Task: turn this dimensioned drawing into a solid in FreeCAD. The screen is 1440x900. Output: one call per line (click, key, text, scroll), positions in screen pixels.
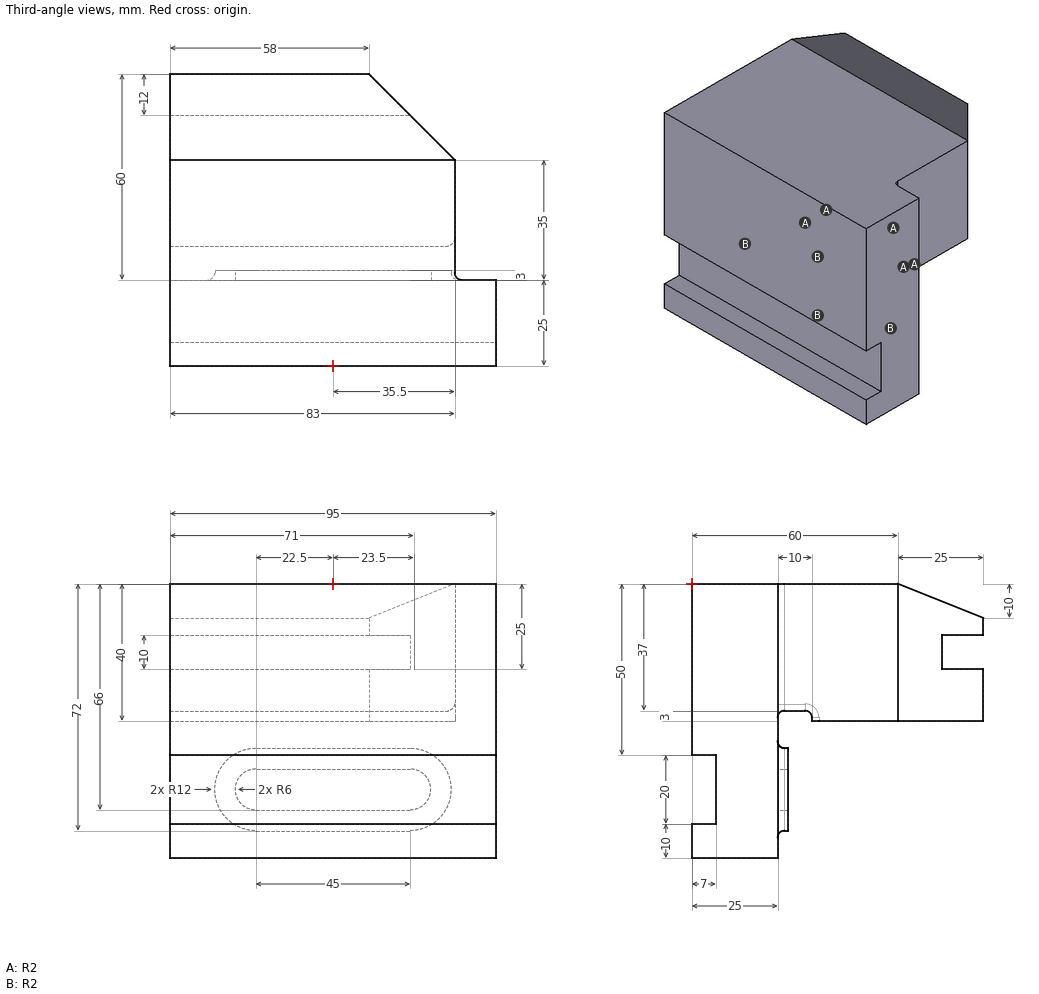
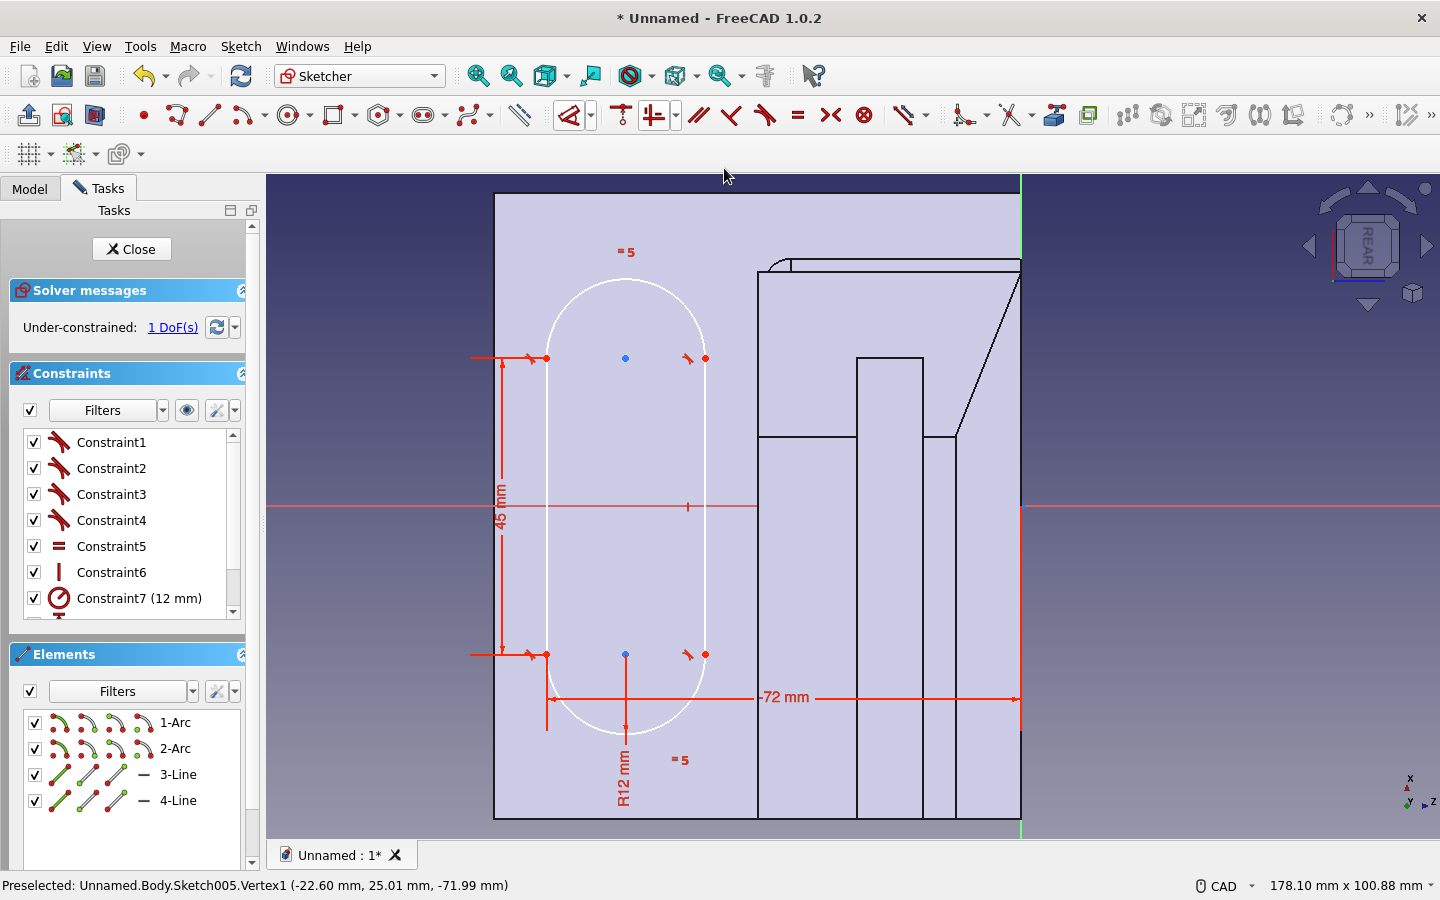
click(547, 655)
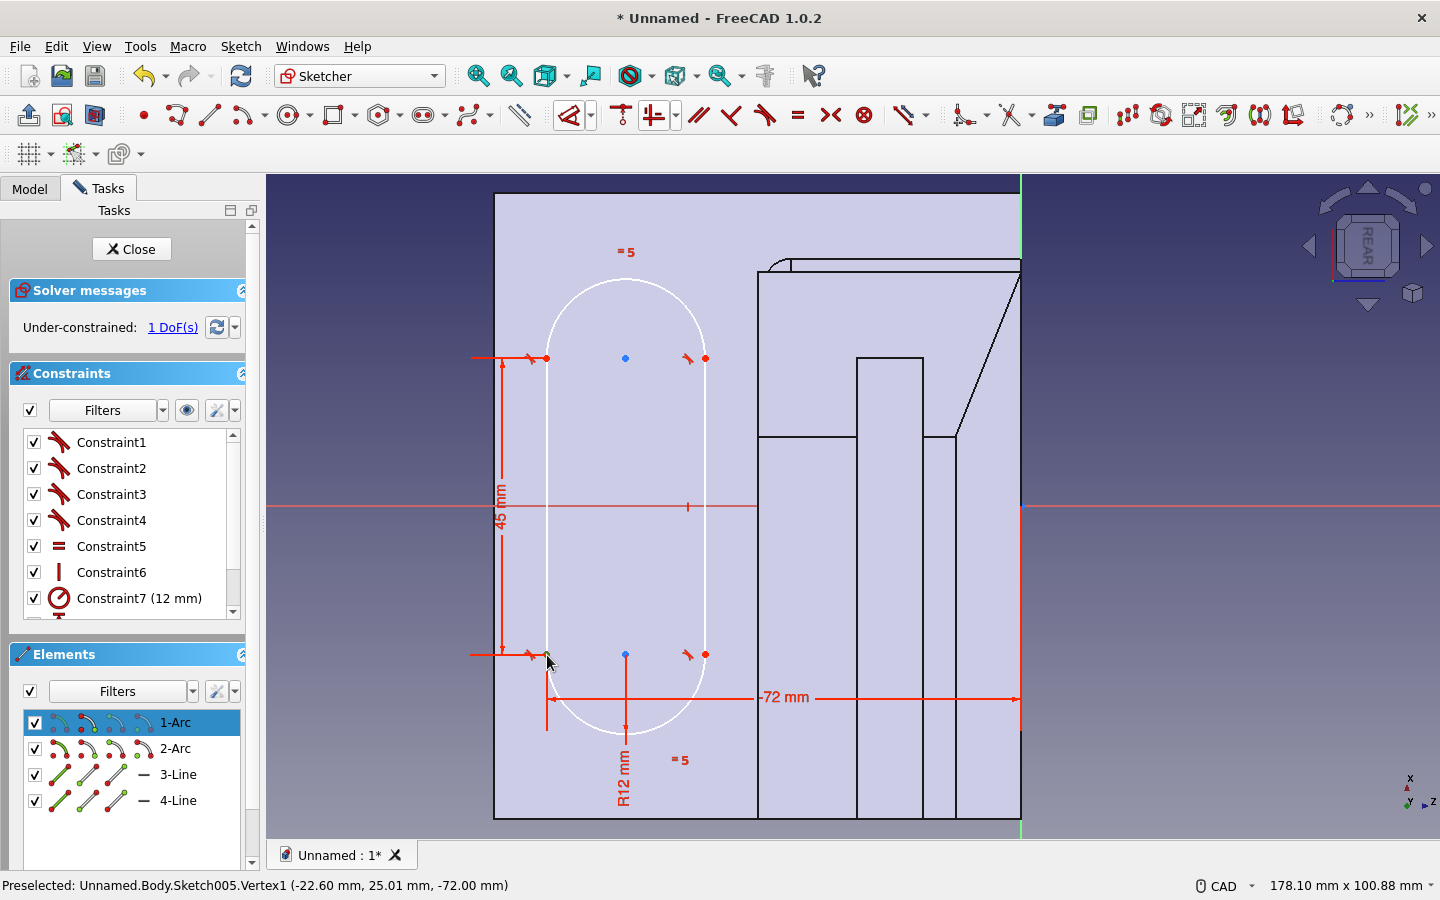
click(590, 116)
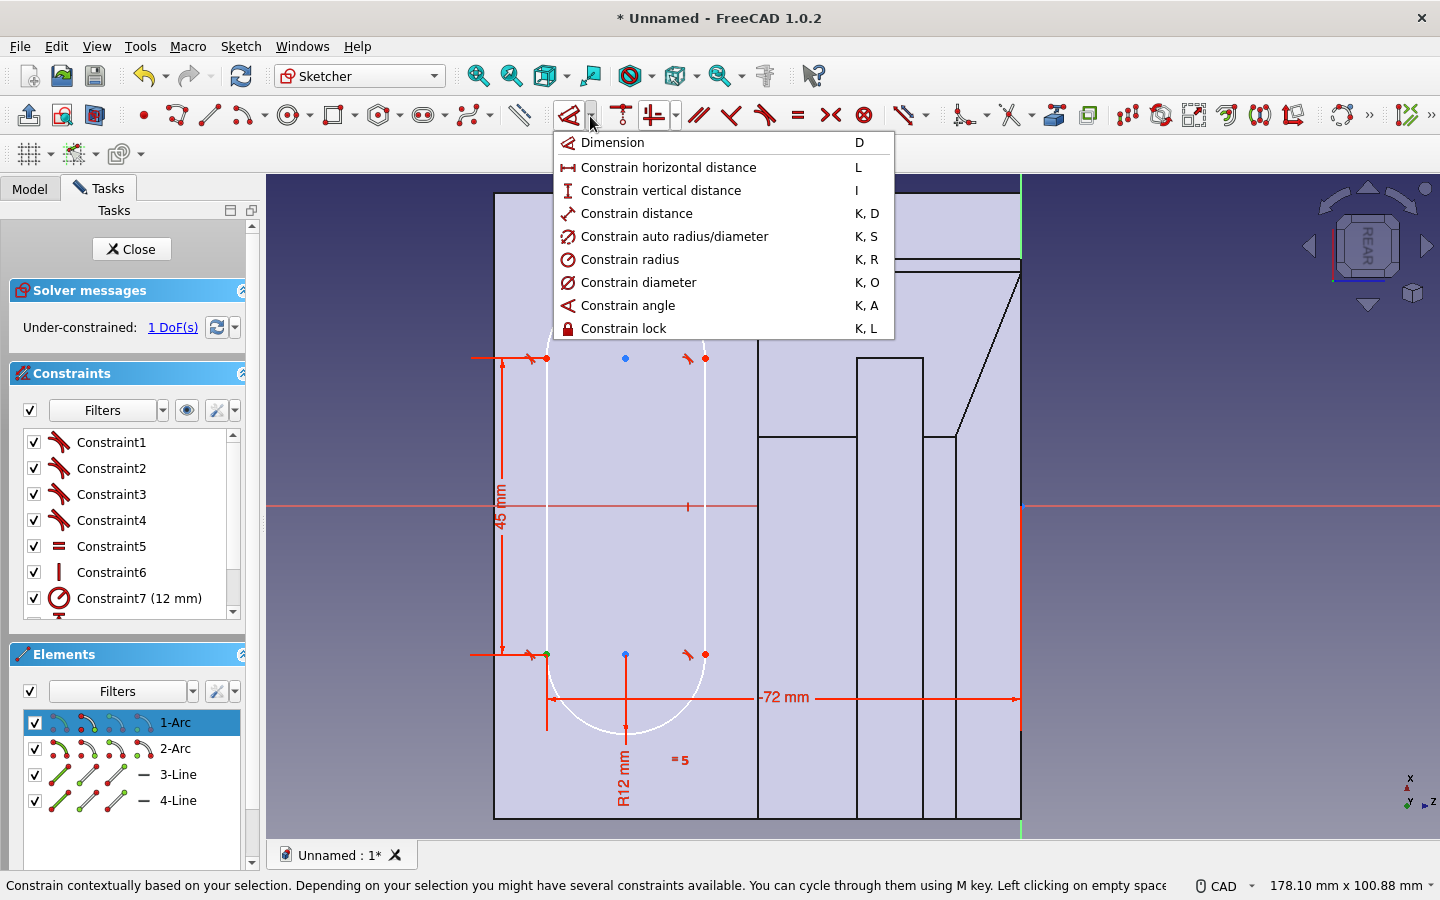
click(724, 190)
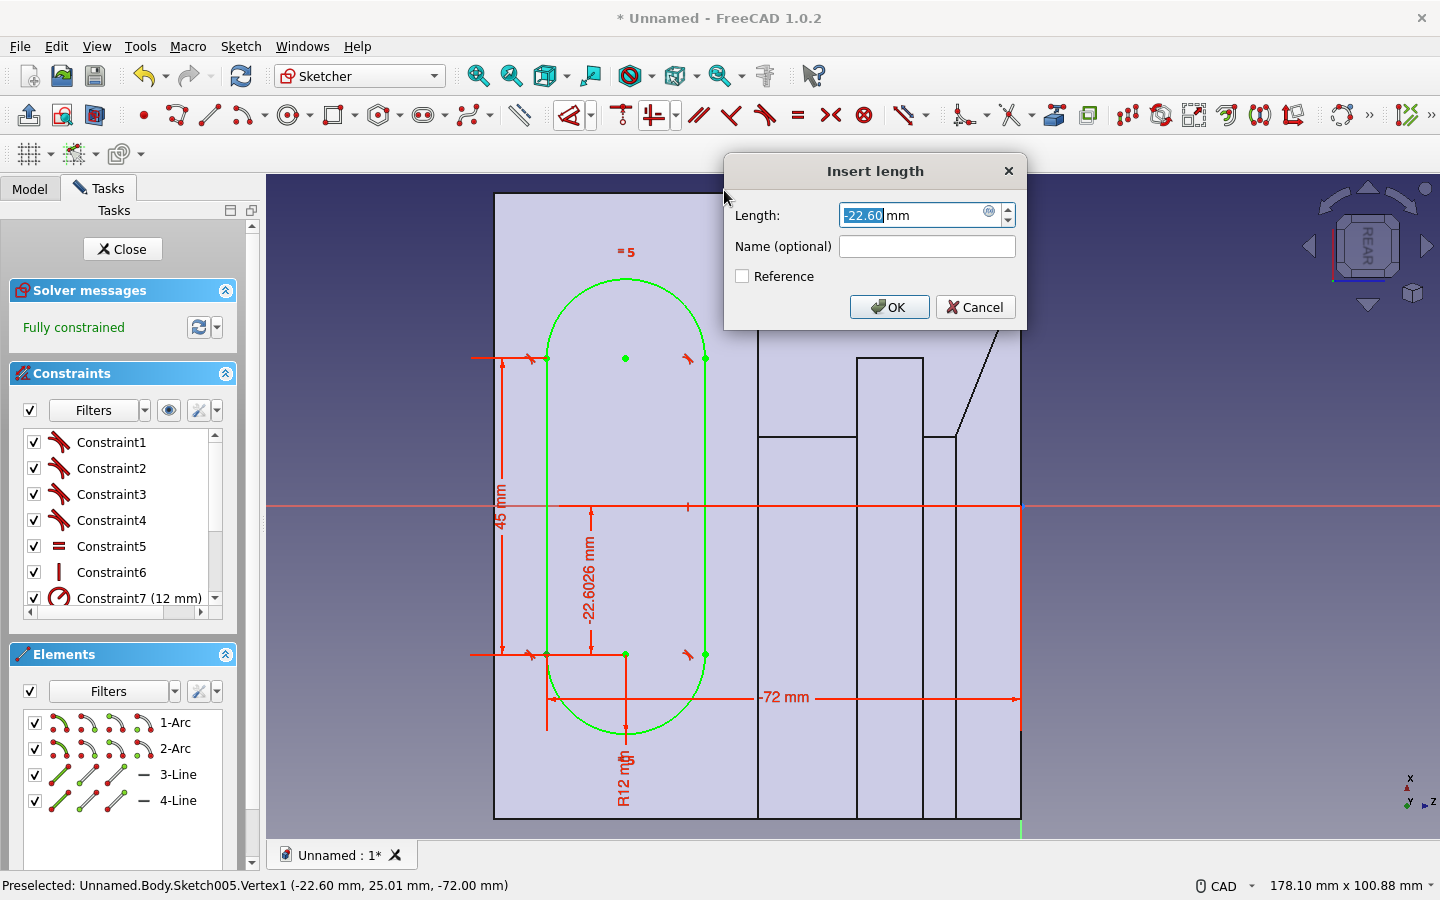
text(-22.5)
key(Return)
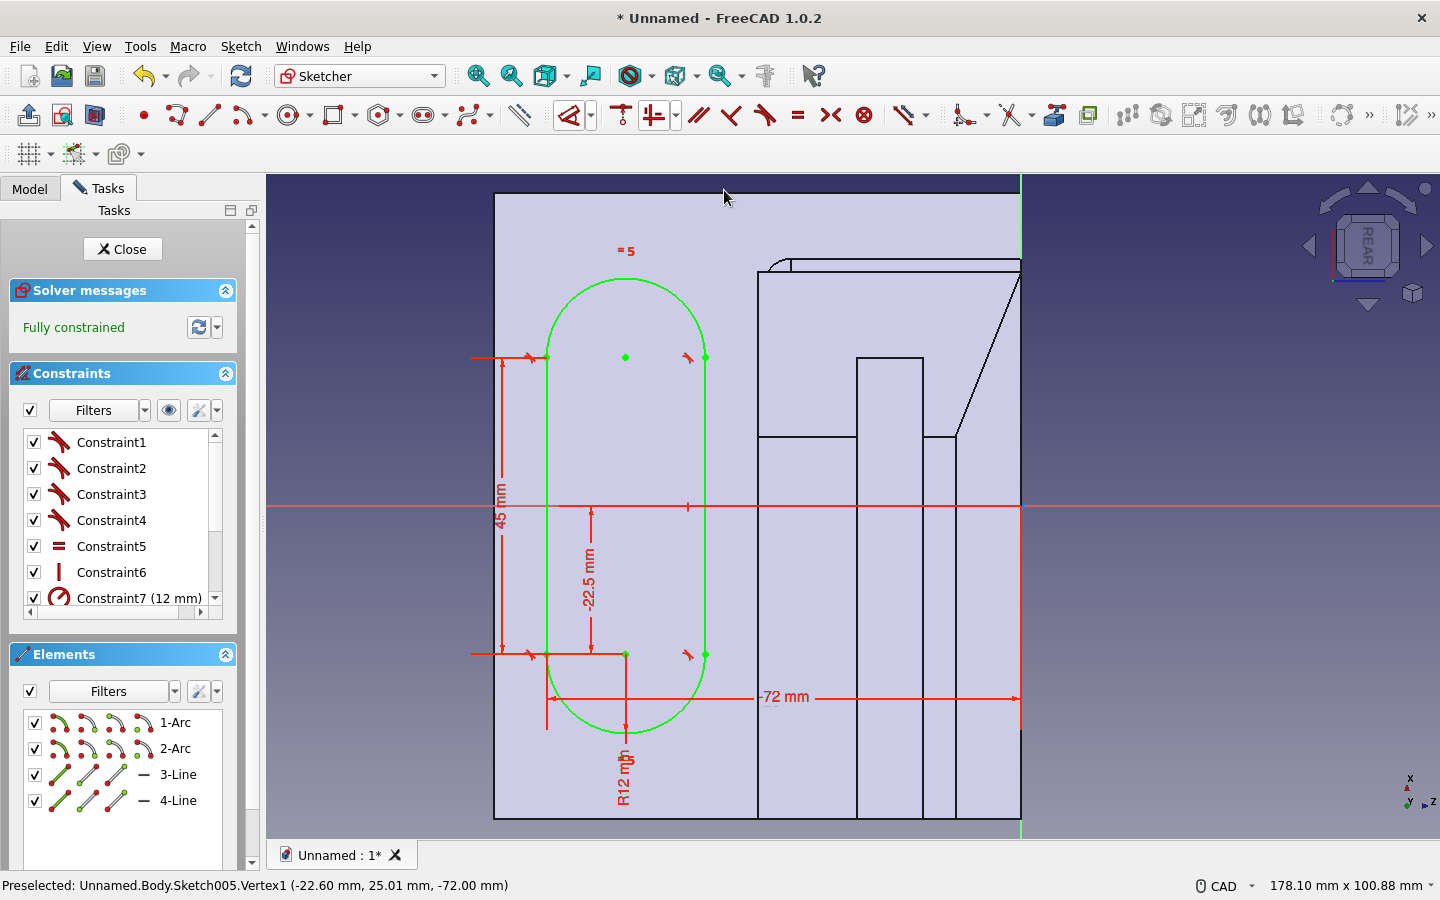
click(123, 249)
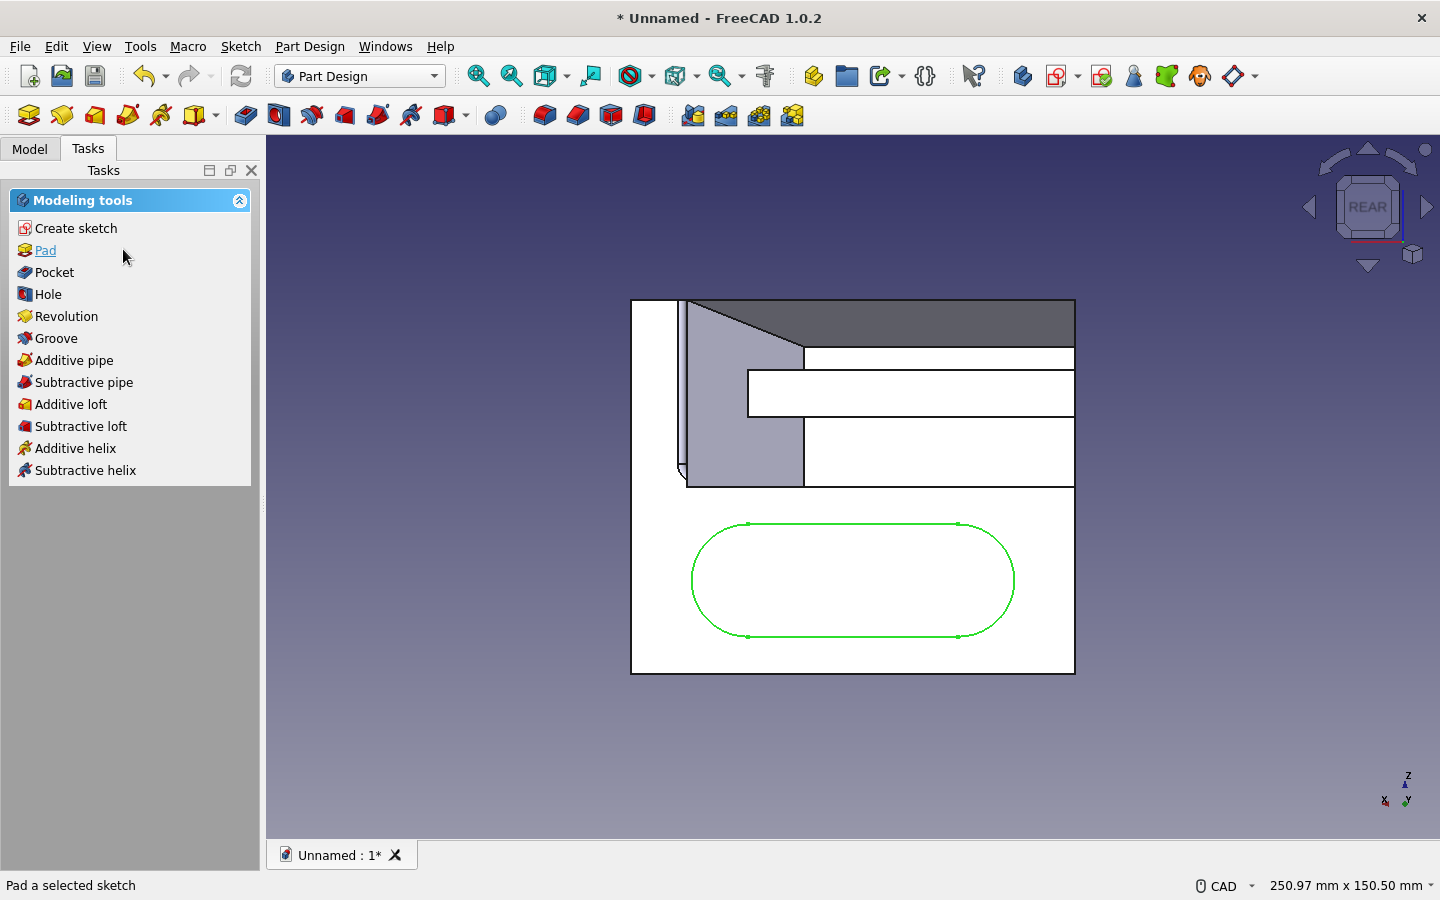
click(29, 116)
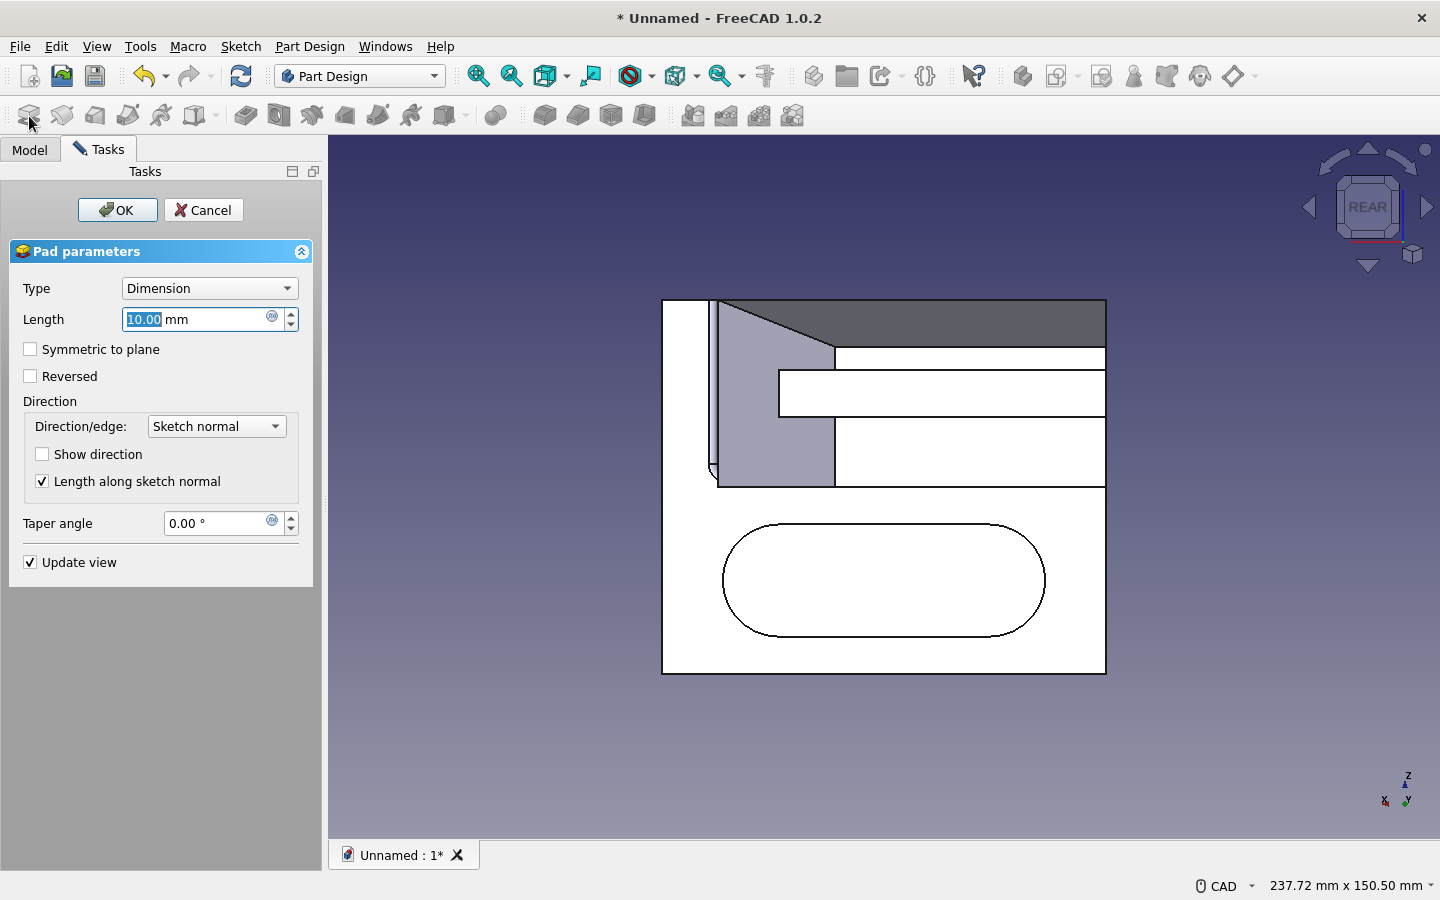
text(3)
key(Tab)